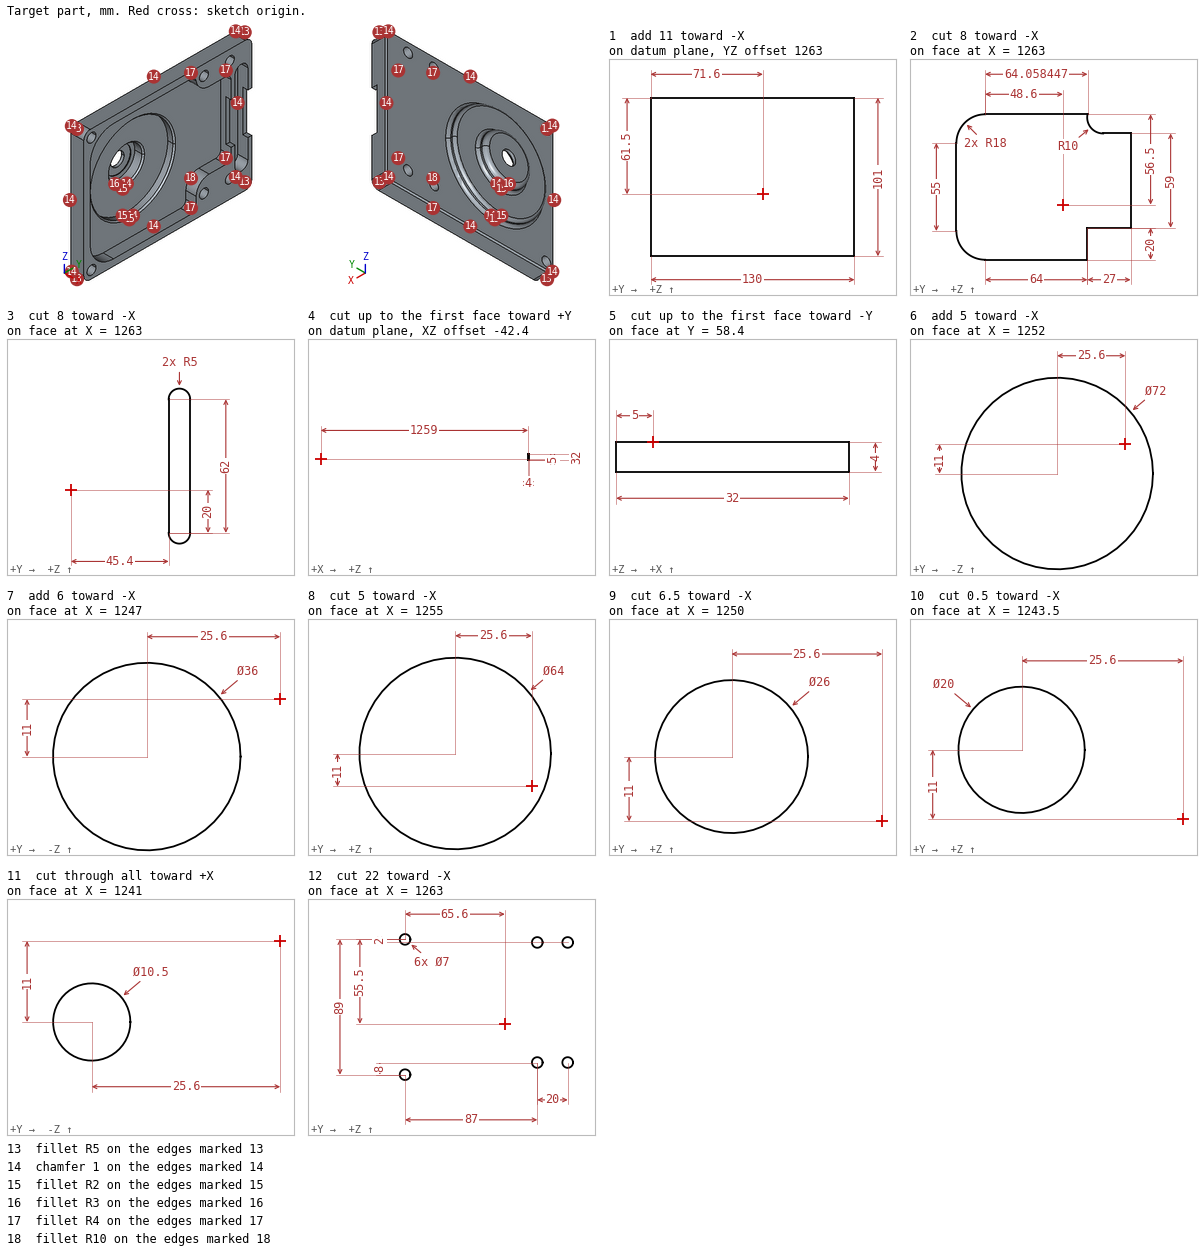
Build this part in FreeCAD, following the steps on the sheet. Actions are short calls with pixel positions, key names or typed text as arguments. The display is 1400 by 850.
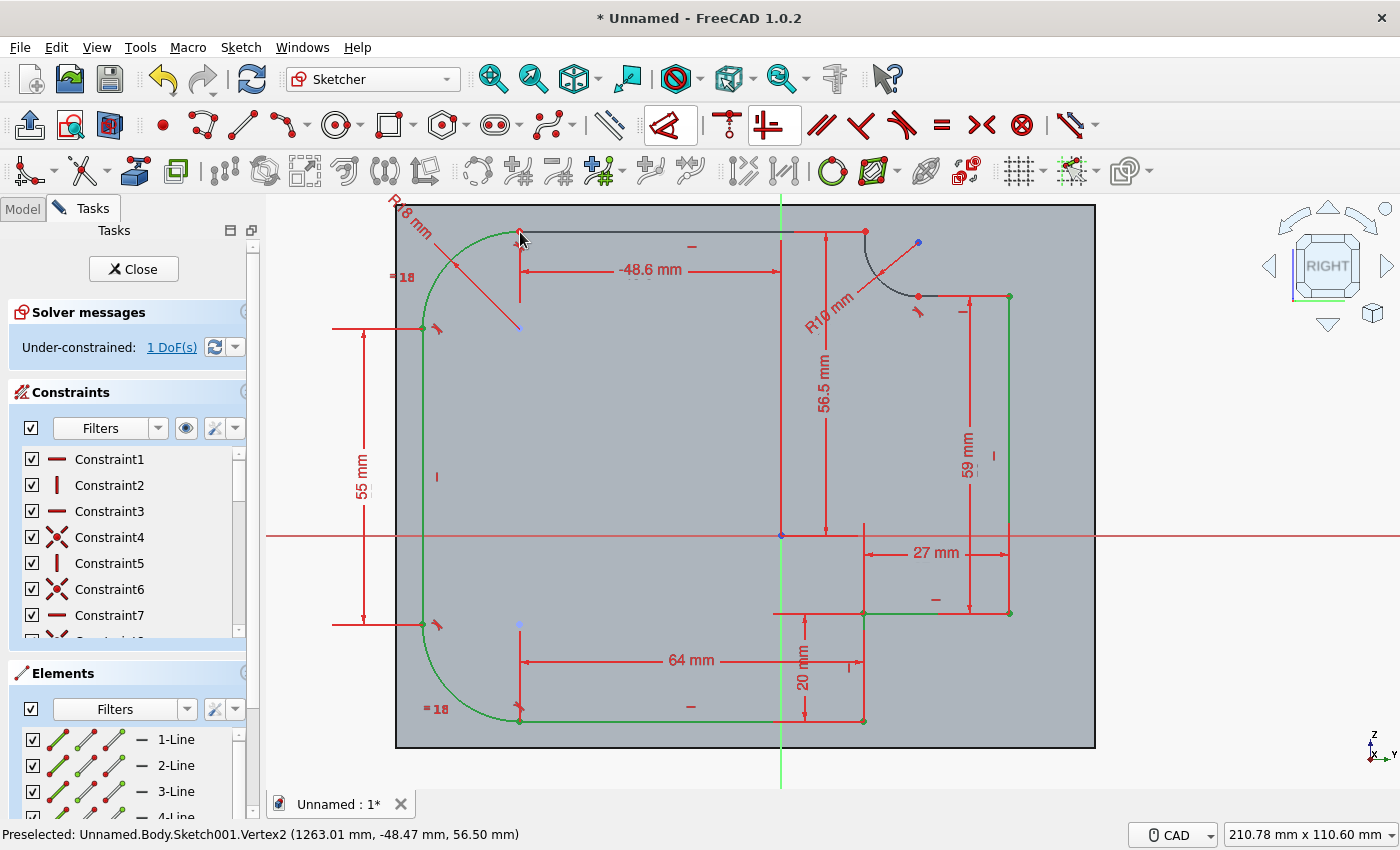
click(762, 232)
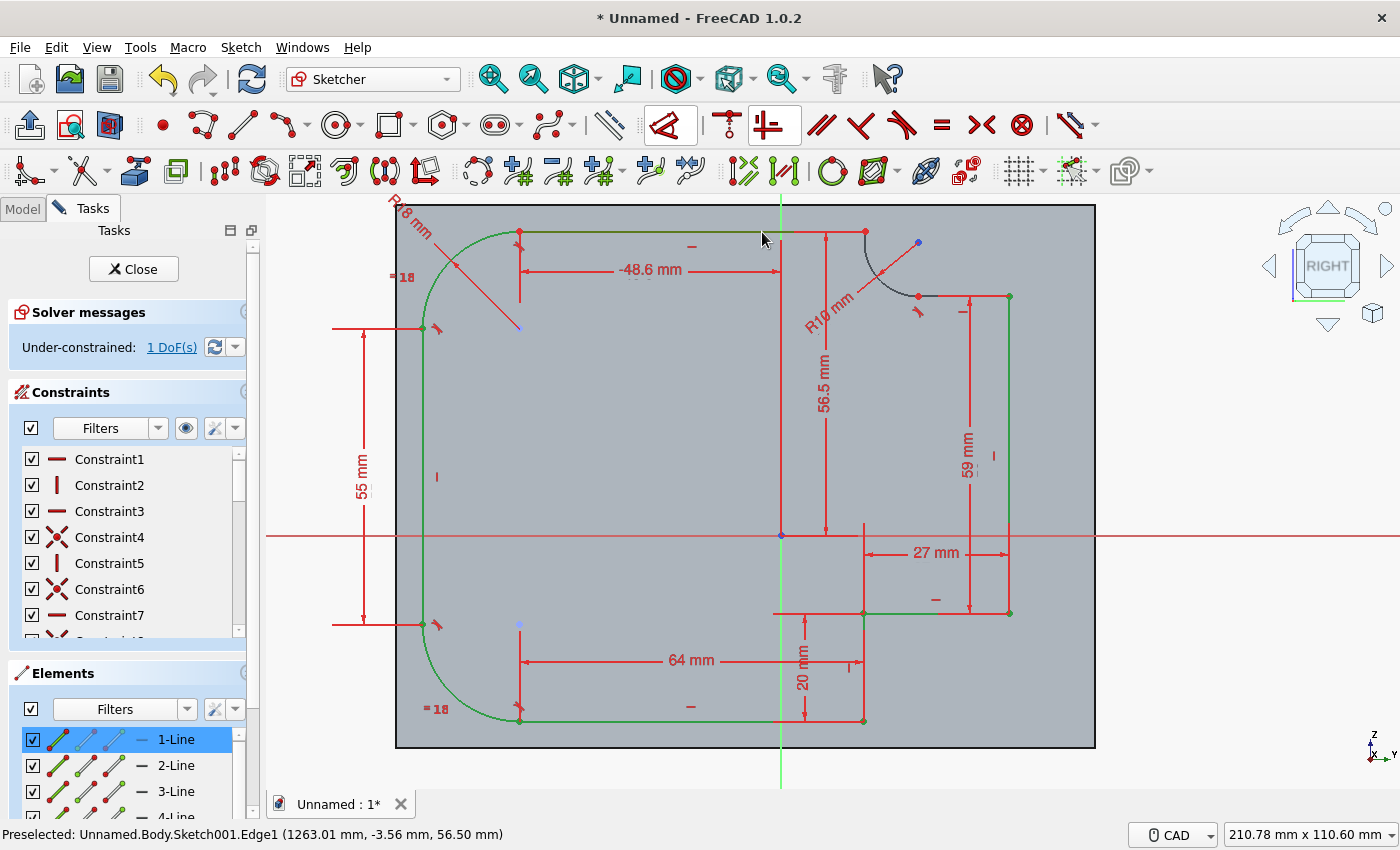
key(l)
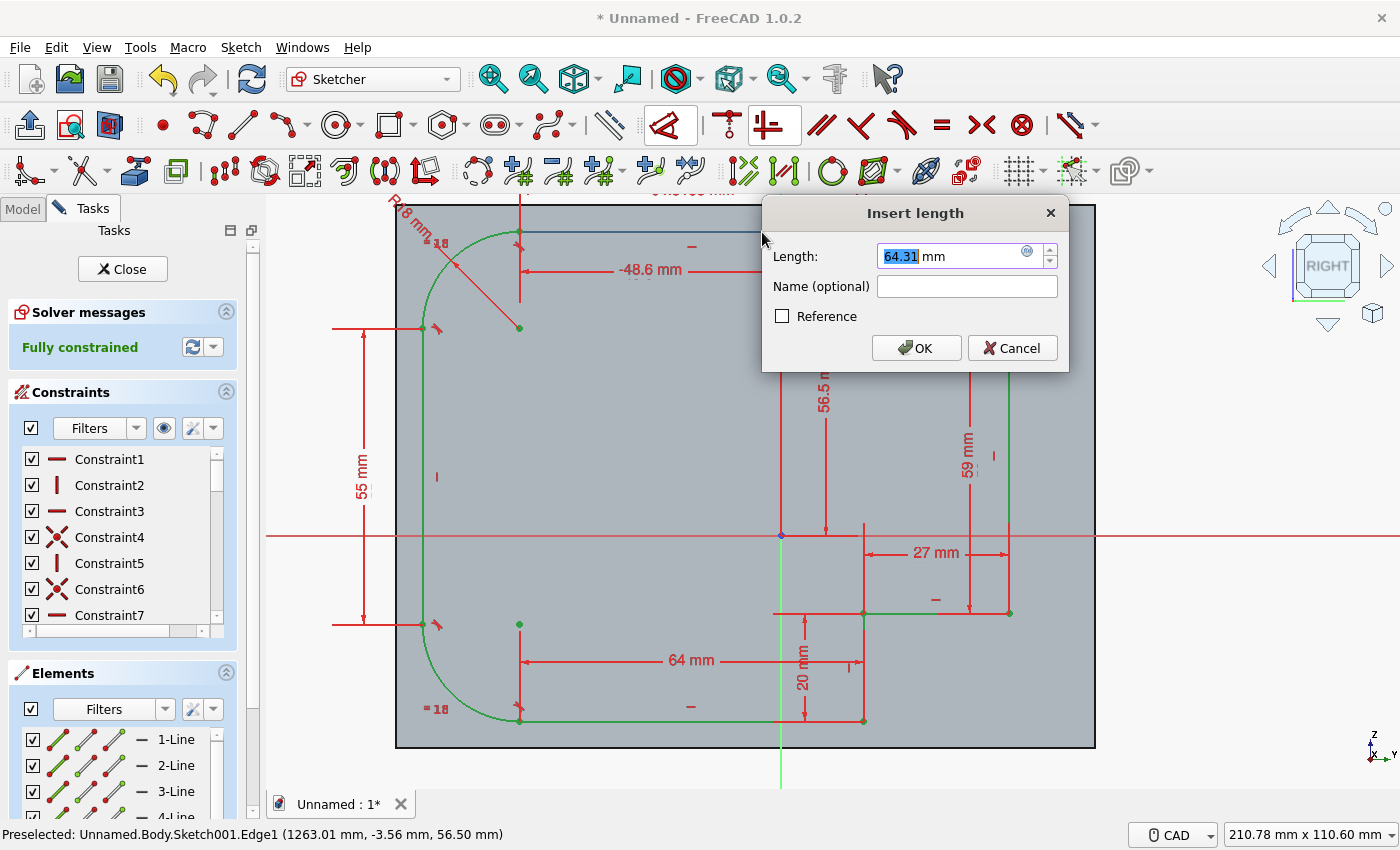
text(64.058447)
key(Return)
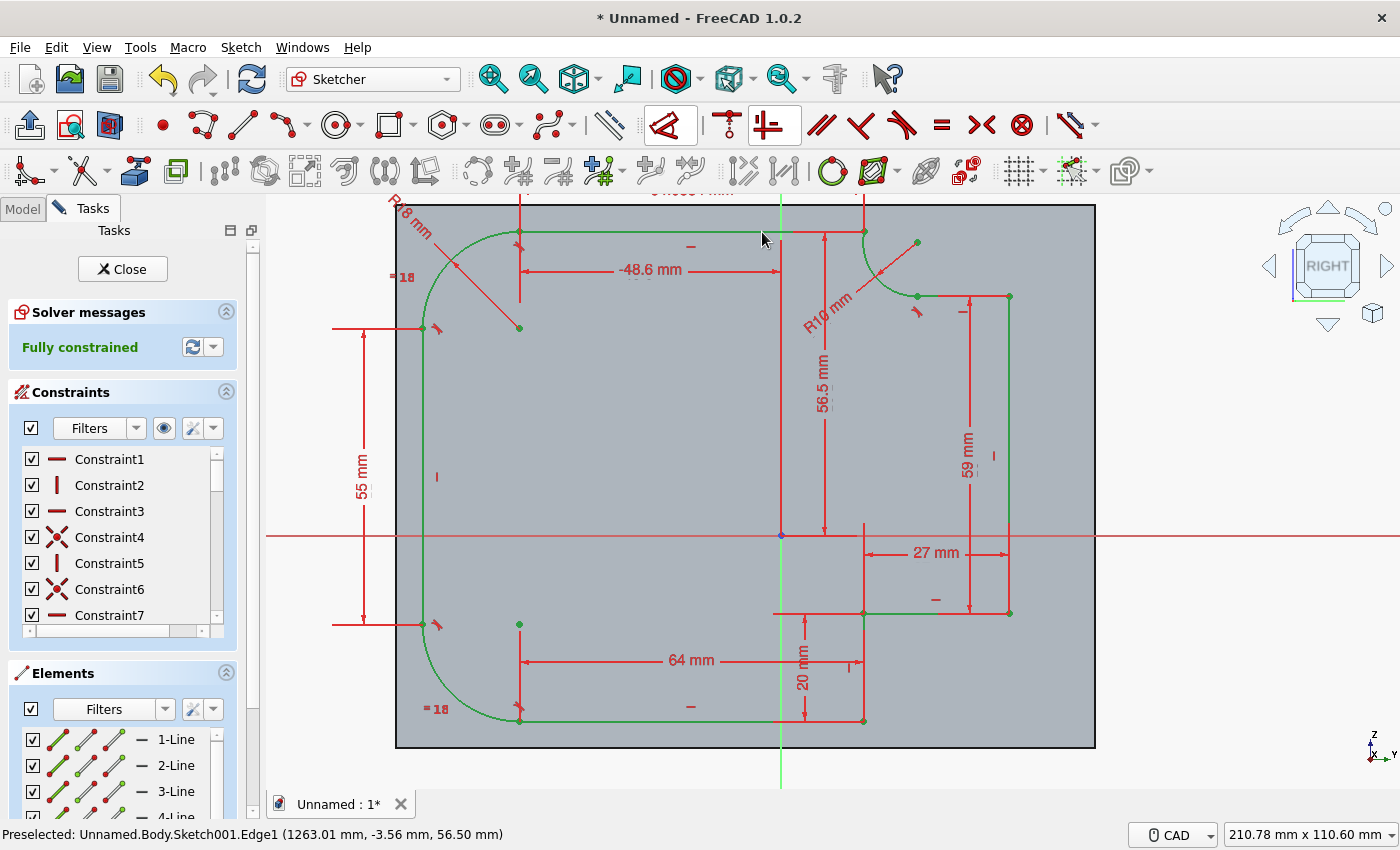
click(123, 269)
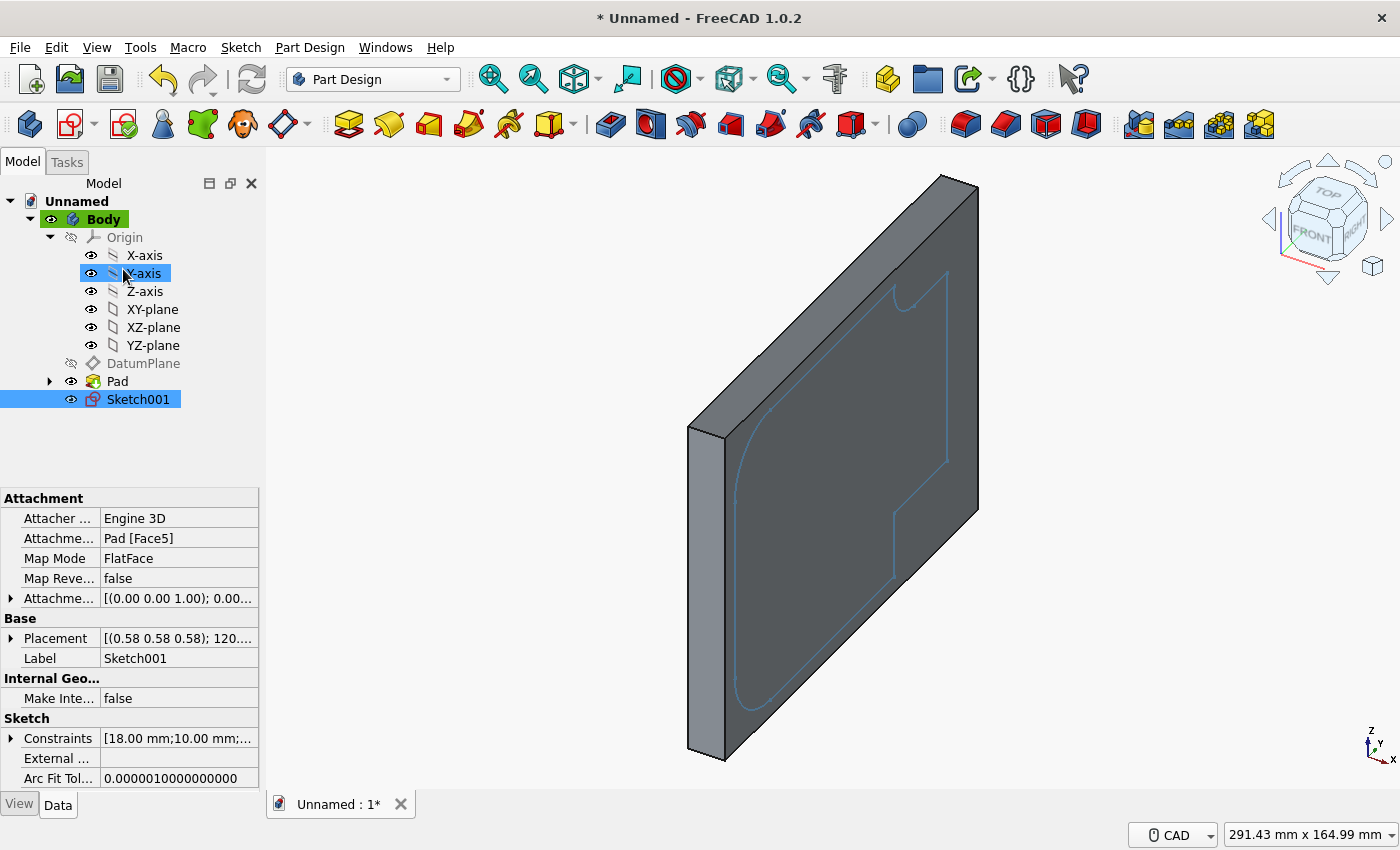
click(612, 124)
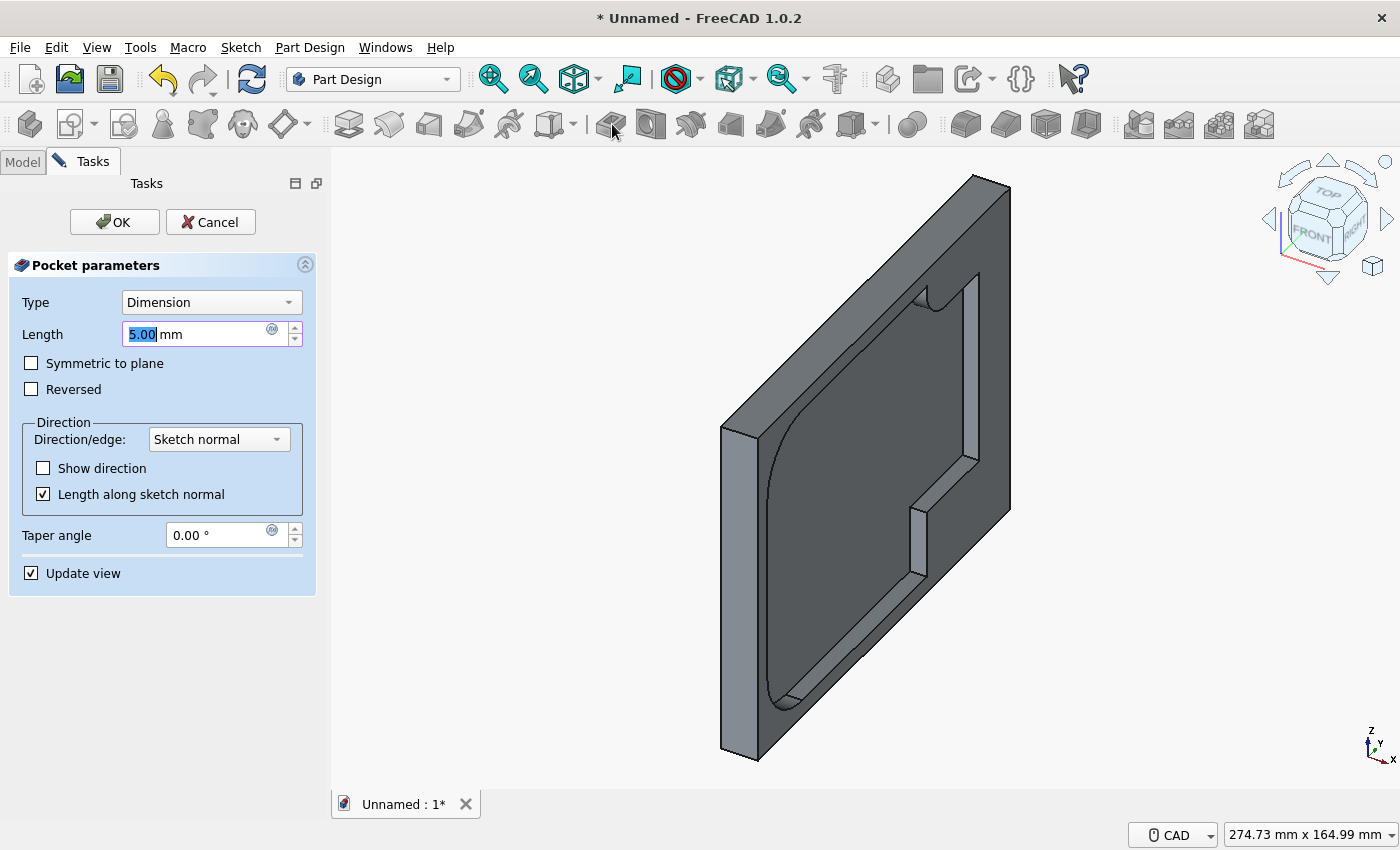
text(8)
key(Tab)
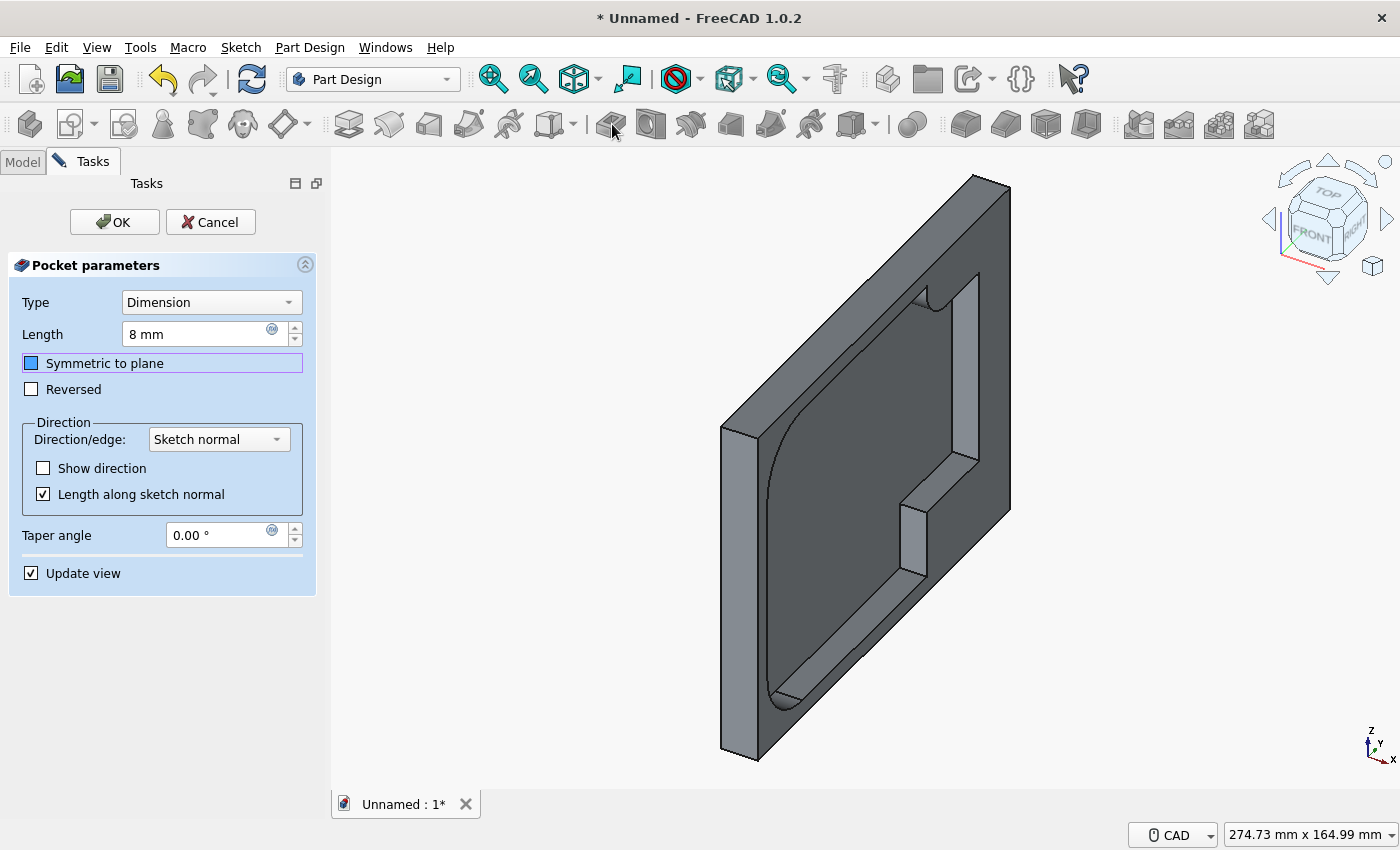
click(115, 222)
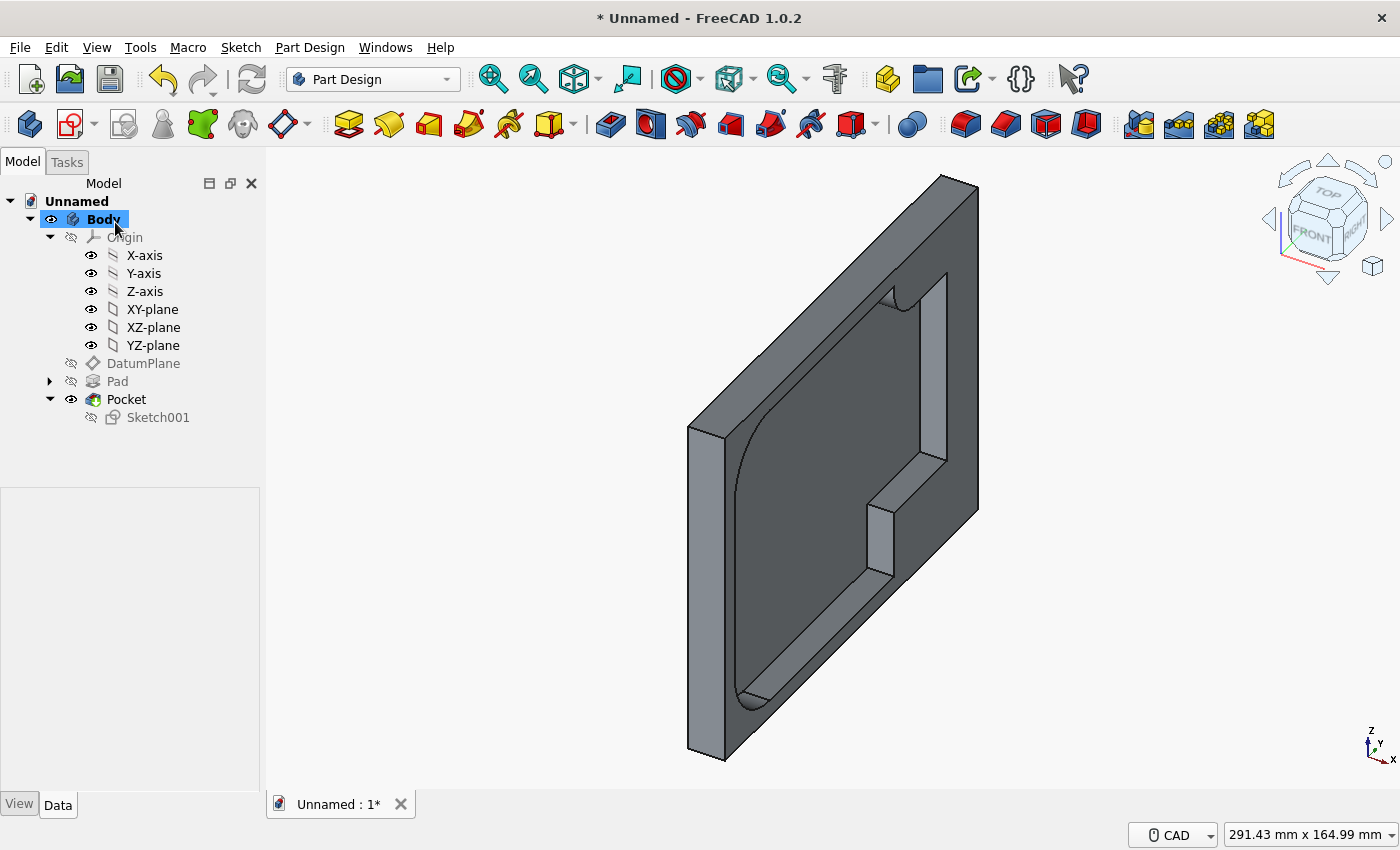
click(960, 457)